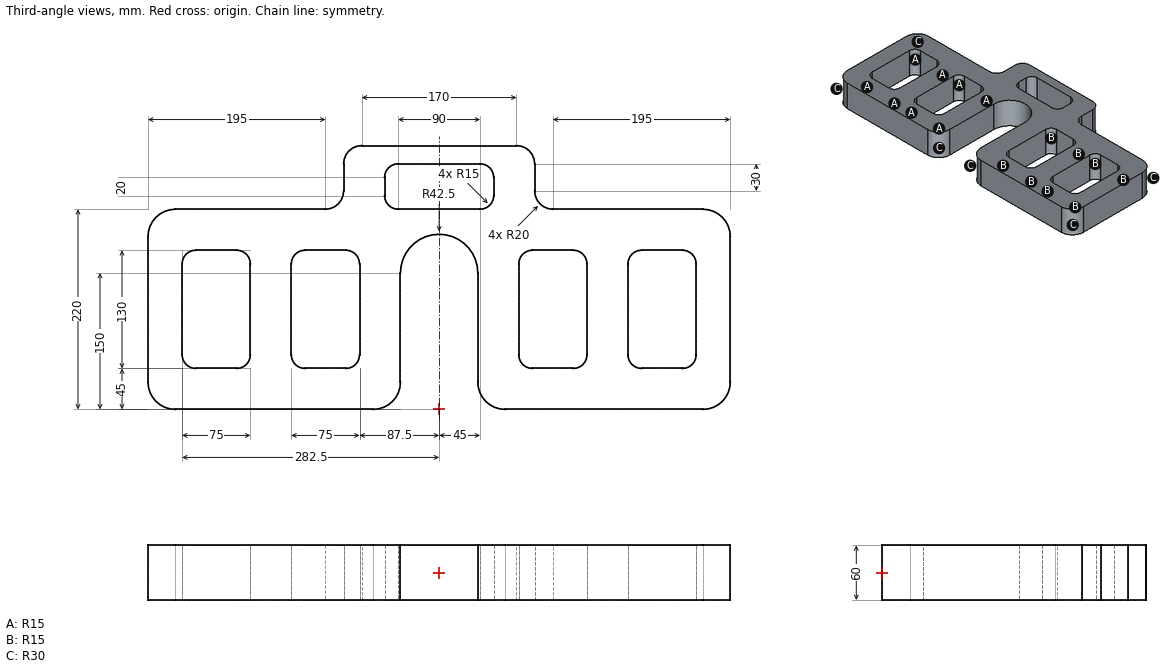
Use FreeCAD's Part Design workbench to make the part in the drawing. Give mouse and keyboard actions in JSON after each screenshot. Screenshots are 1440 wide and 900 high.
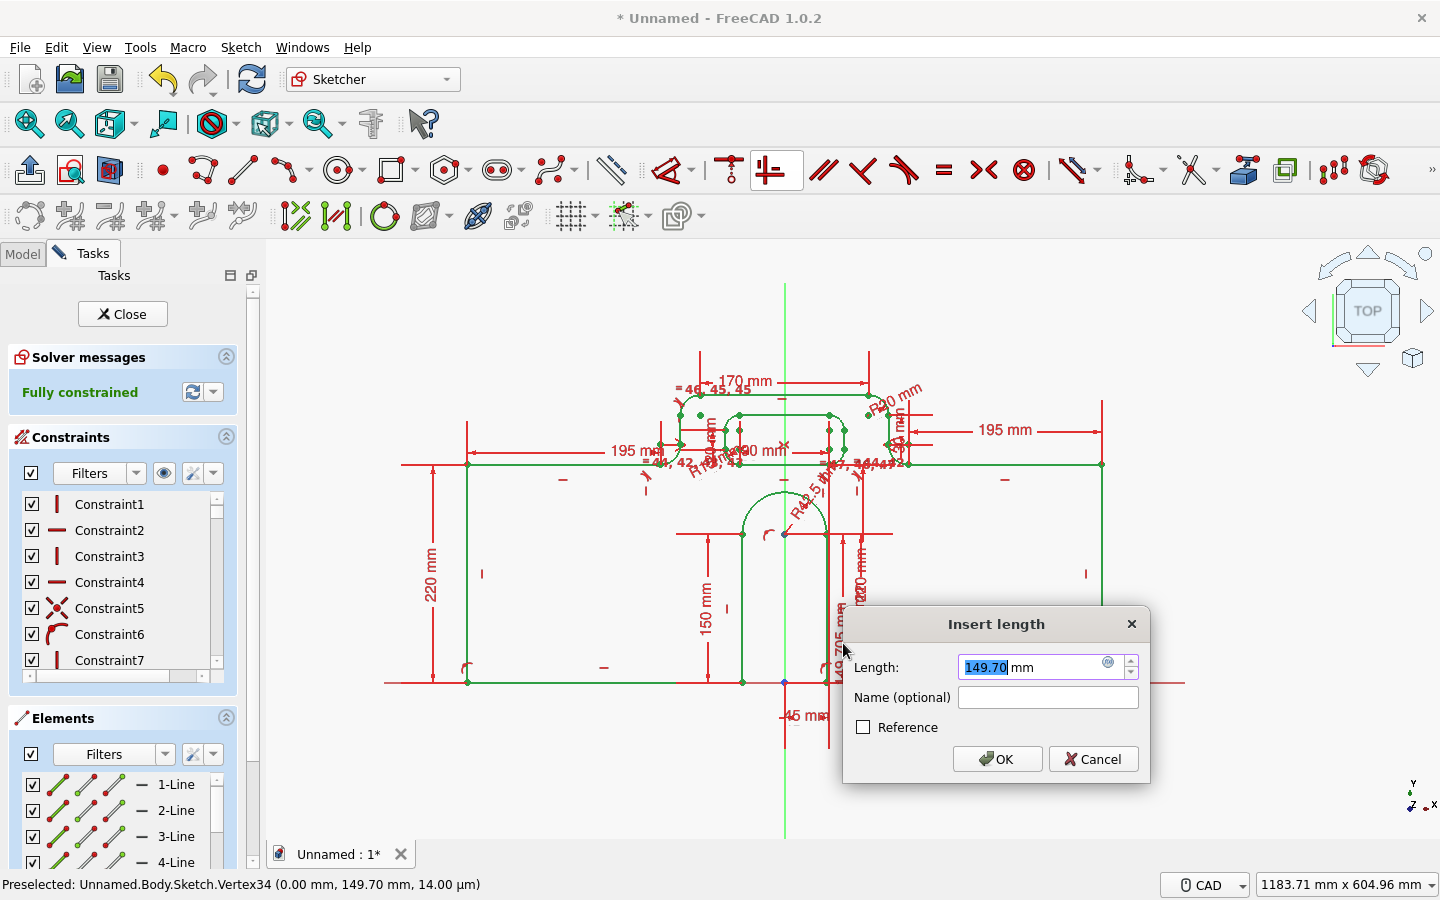
{"action": "type", "text": "150"}
{"action": "key", "text": "Return"}
{"action": "key", "text": "Escape"}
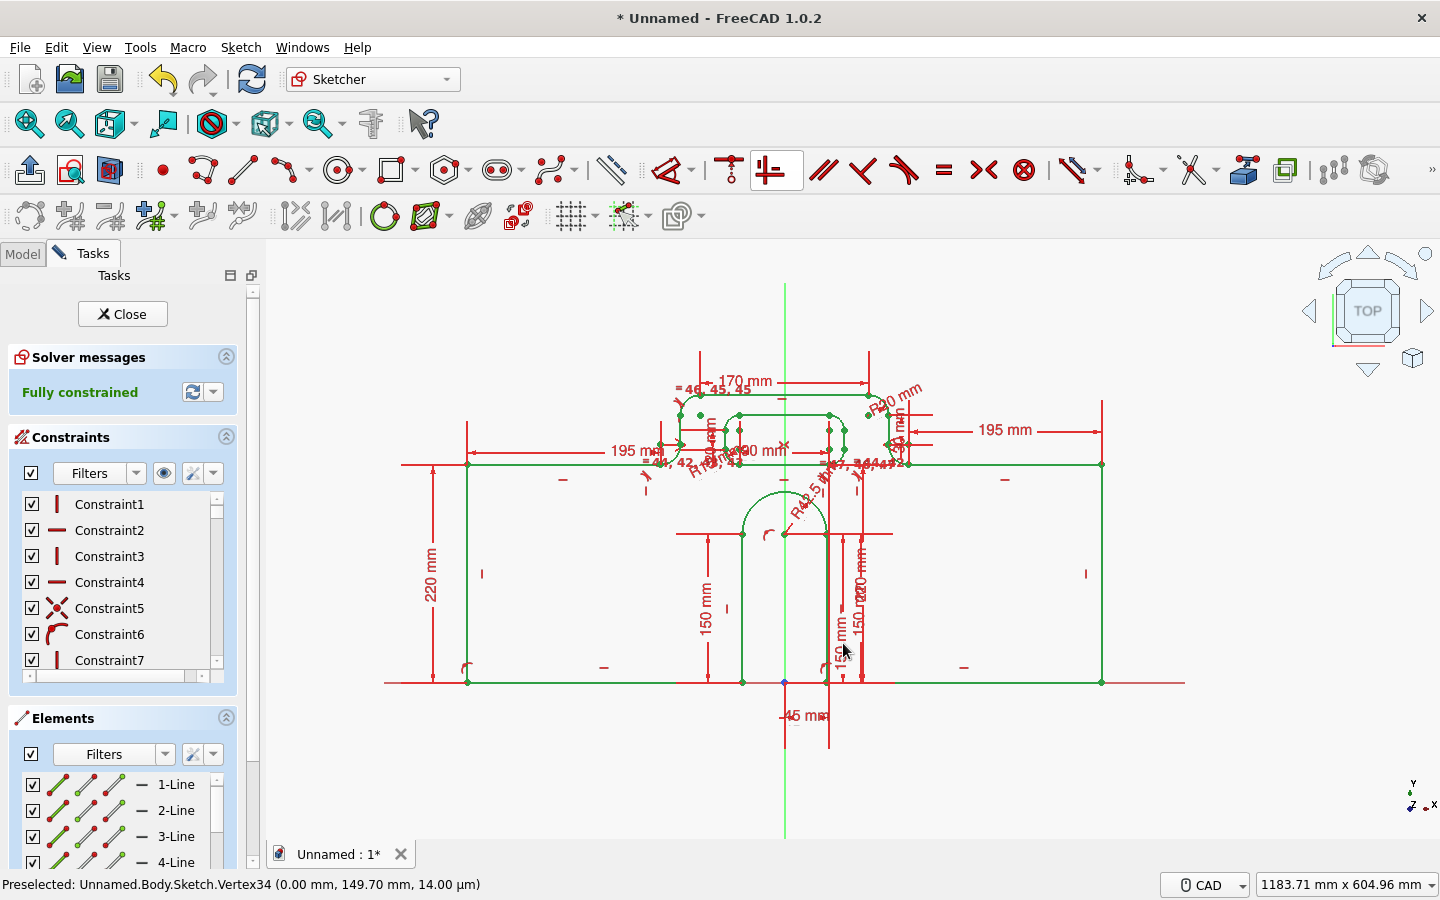
{"action": "left_click", "coordinate": [123, 314]}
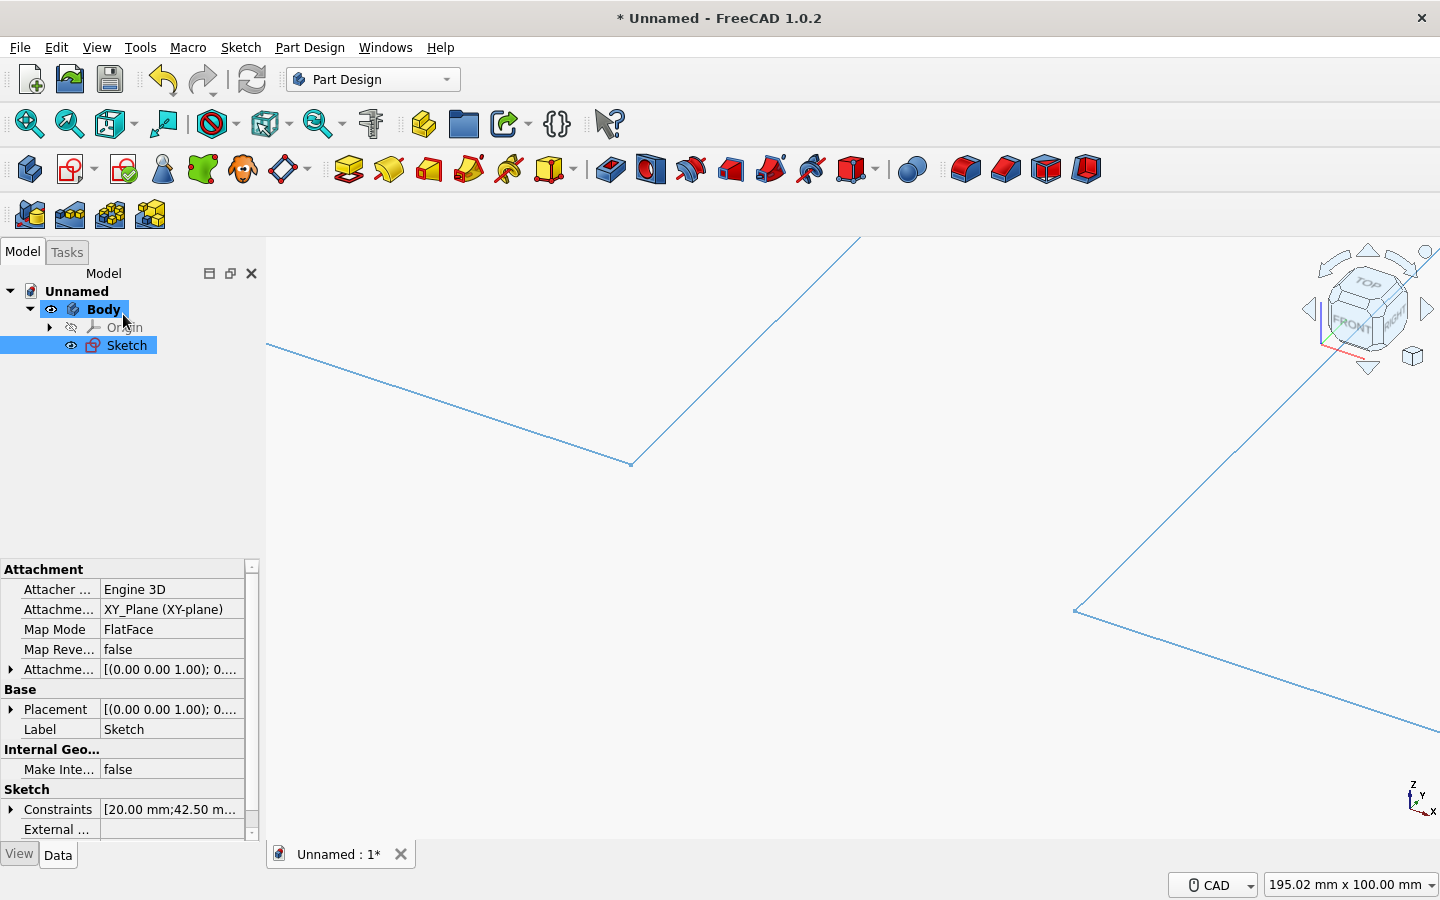
{"action": "left_click", "coordinate": [350, 170]}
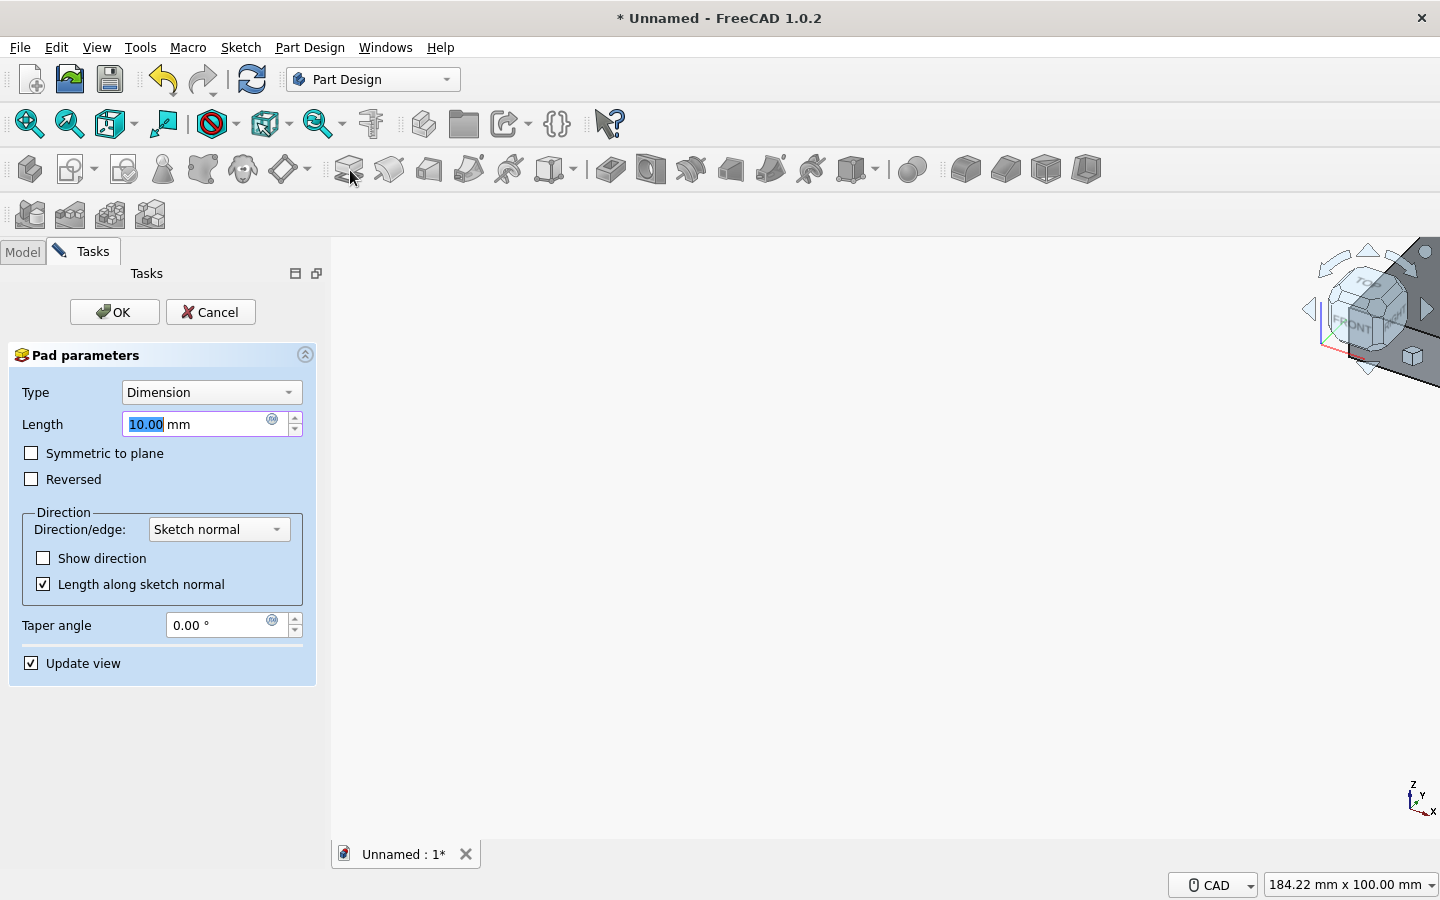
{"action": "type", "text": "60"}
{"action": "key", "text": "Tab"}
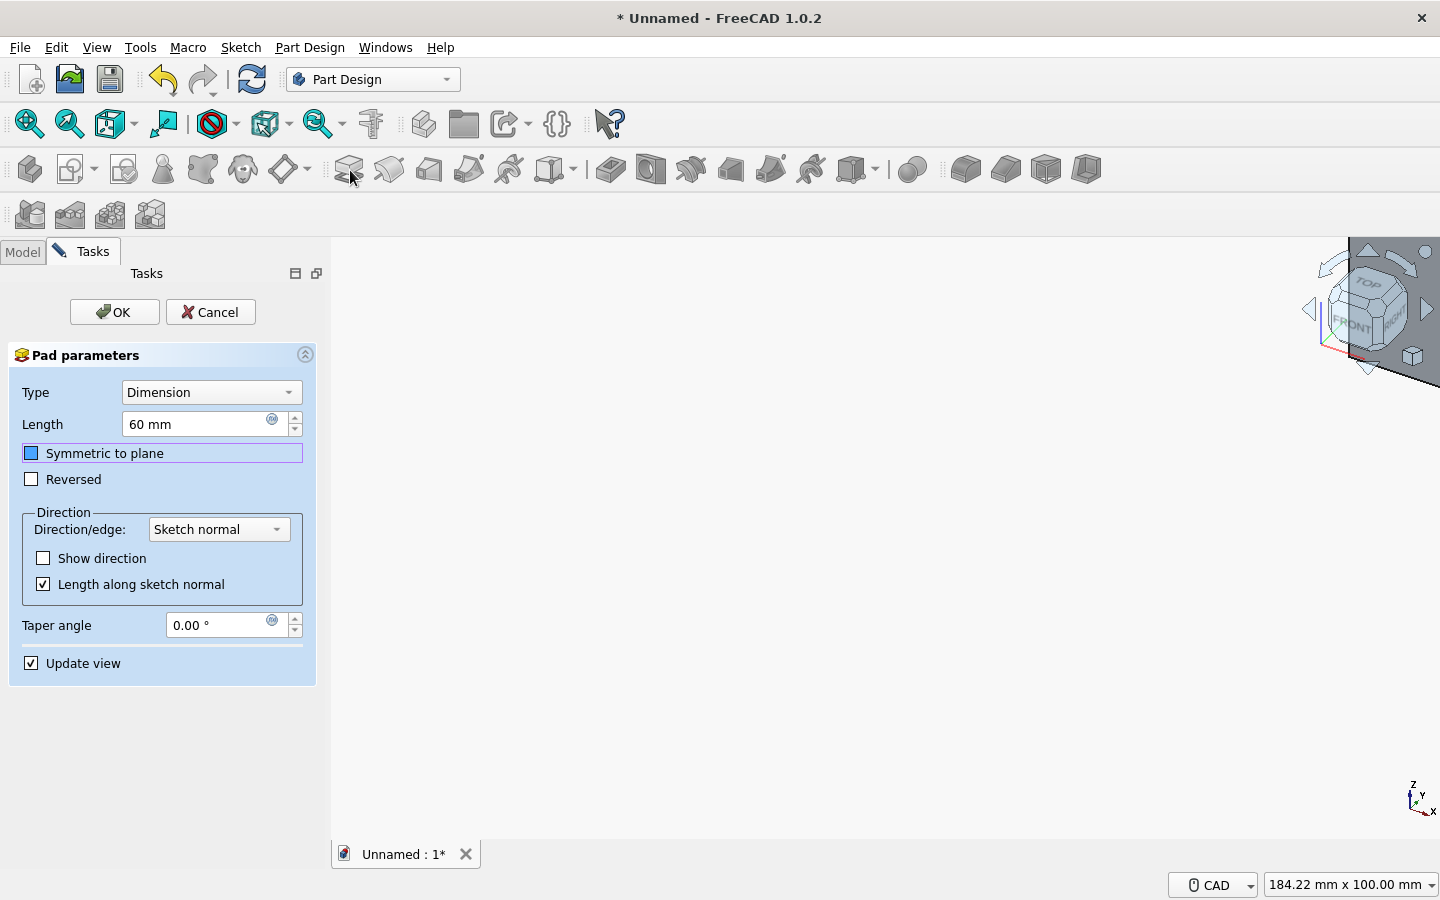
{"action": "left_click", "coordinate": [30, 453]}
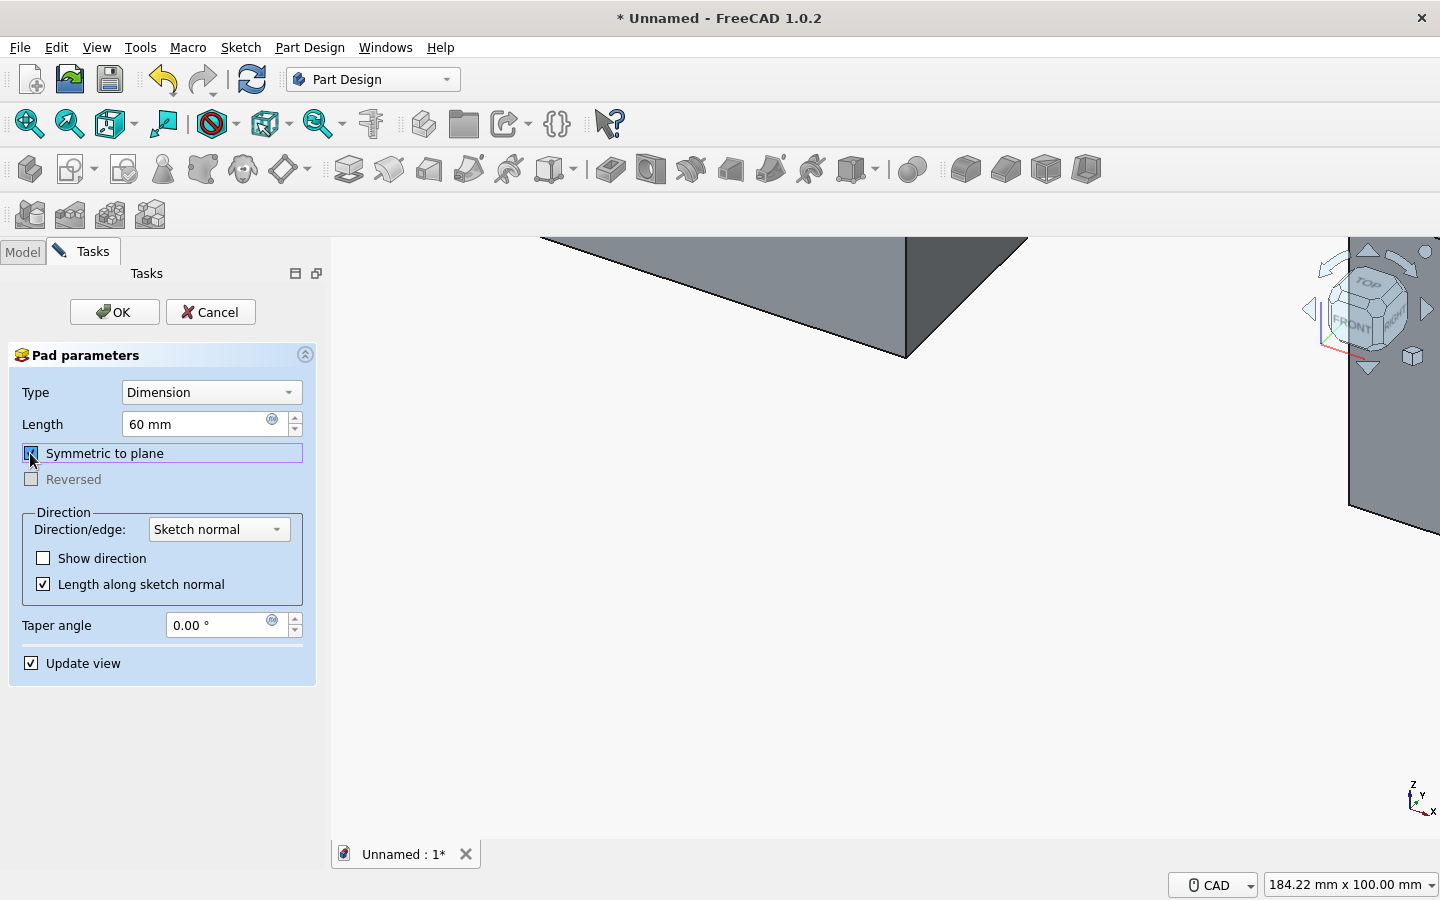
{"action": "left_click", "coordinate": [115, 312]}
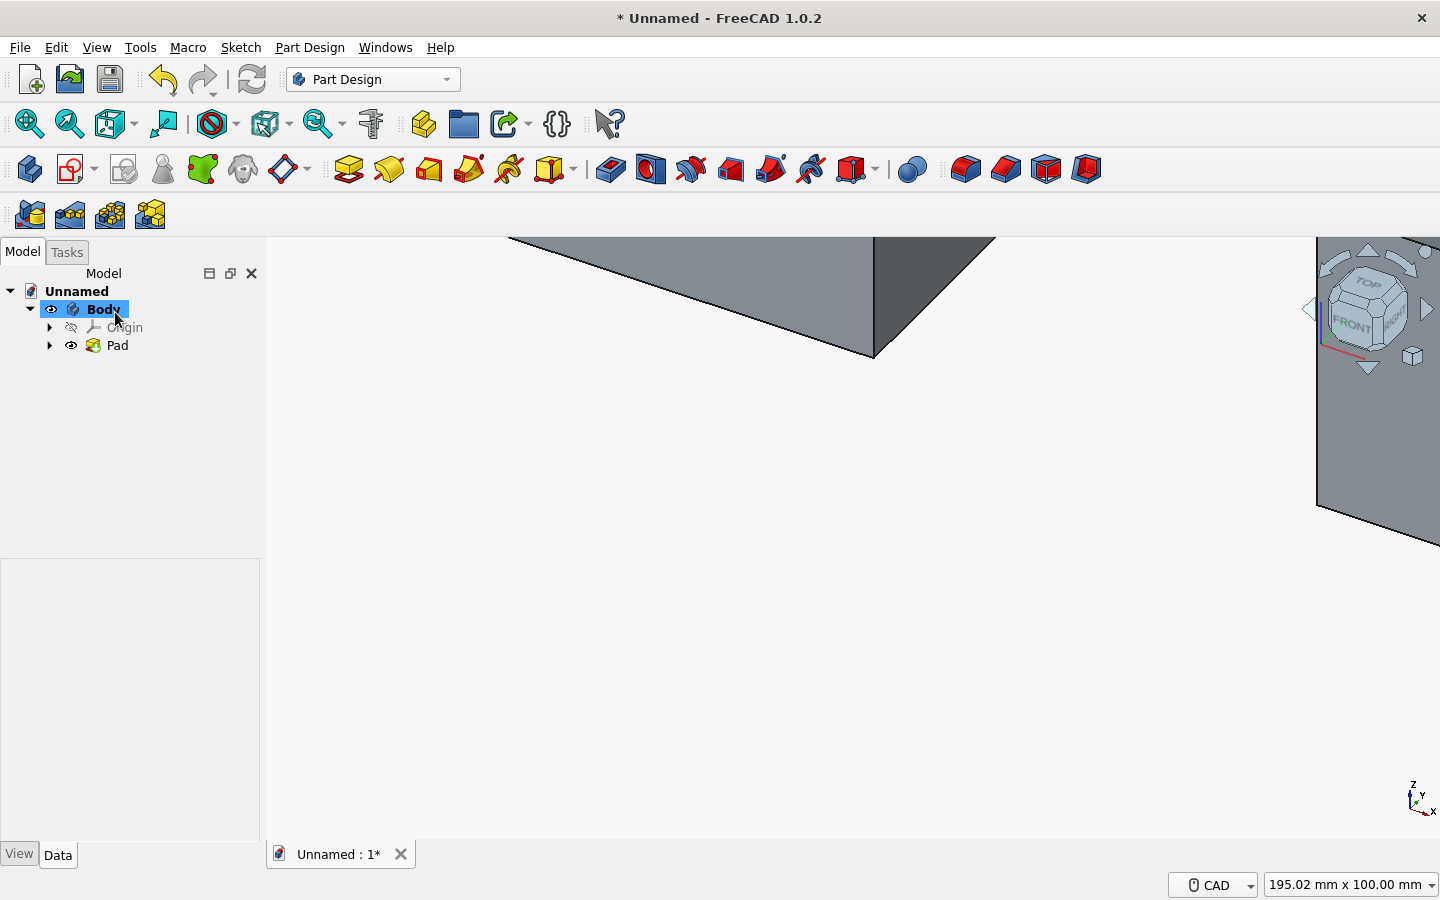
{"action": "key", "text": "v f"}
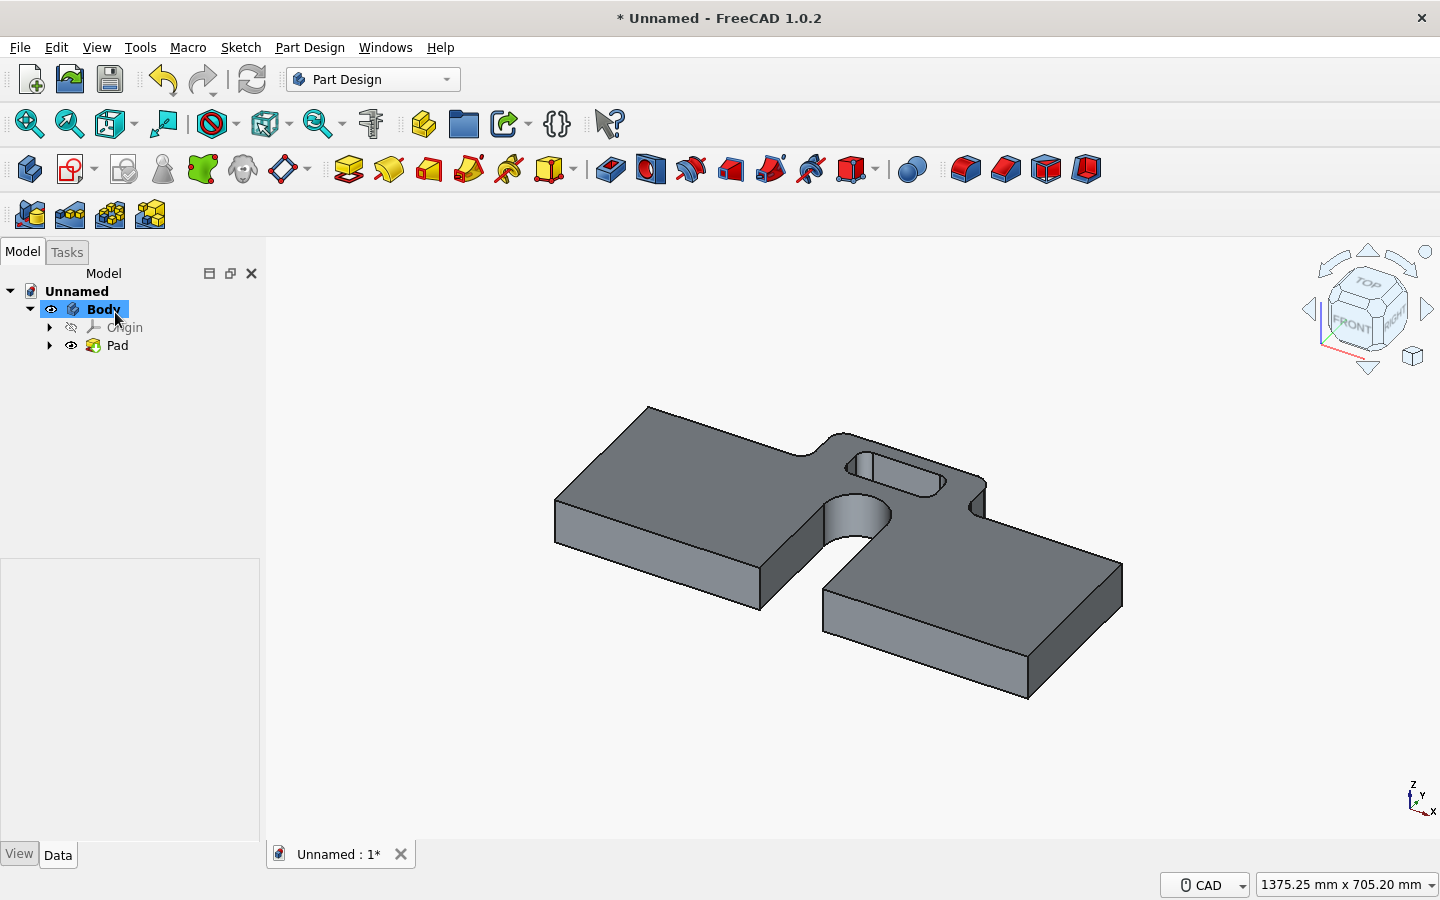
{"action": "left_click", "coordinate": [70, 170]}